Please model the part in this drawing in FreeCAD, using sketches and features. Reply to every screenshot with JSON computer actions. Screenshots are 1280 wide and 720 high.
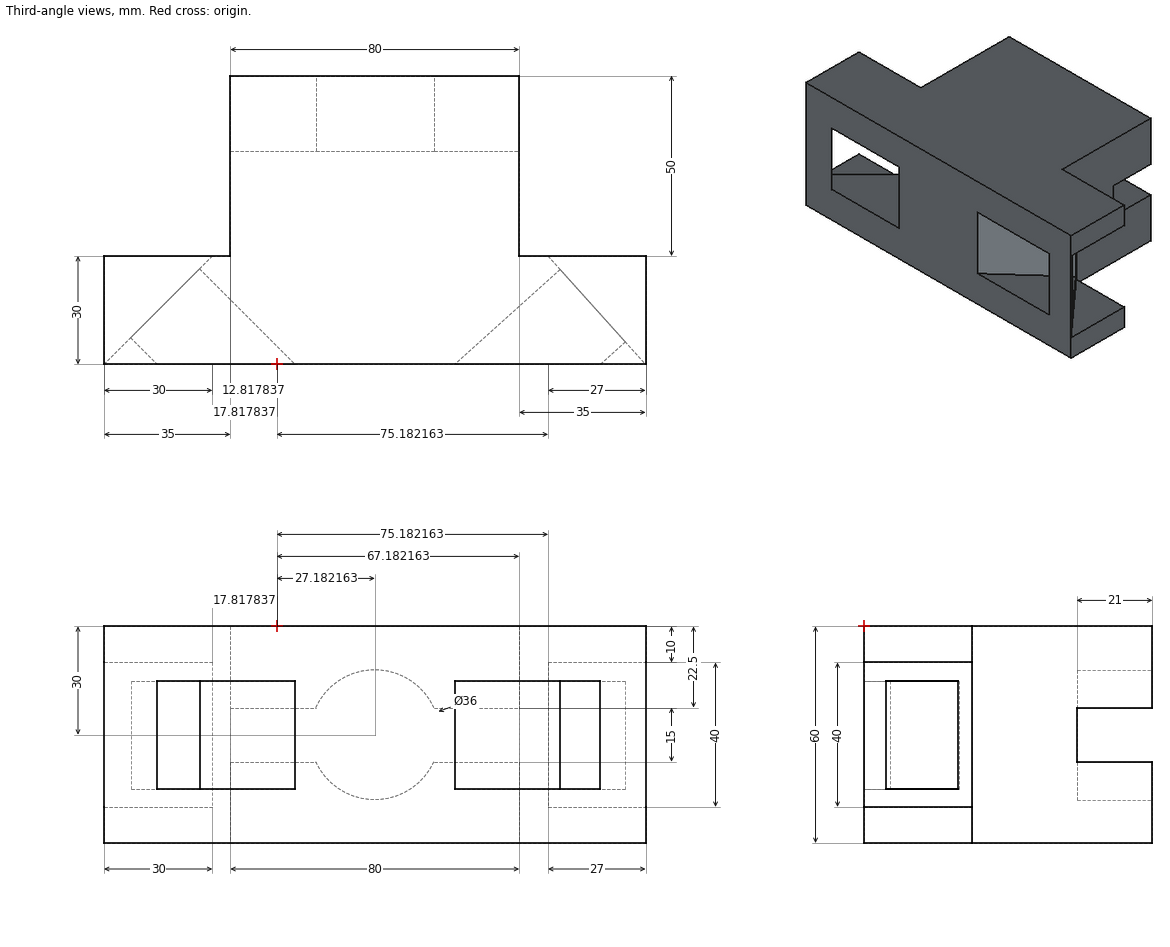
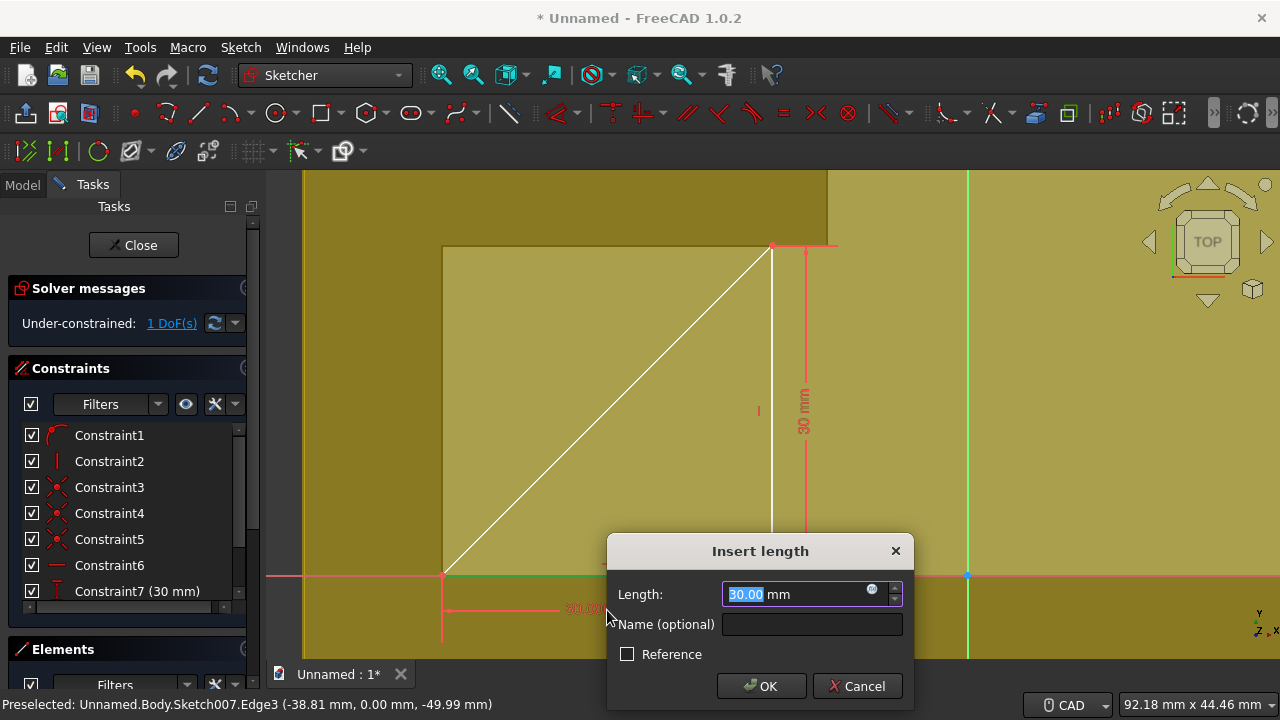
{"action": "type", "text": "30"}
{"action": "key", "text": "Return"}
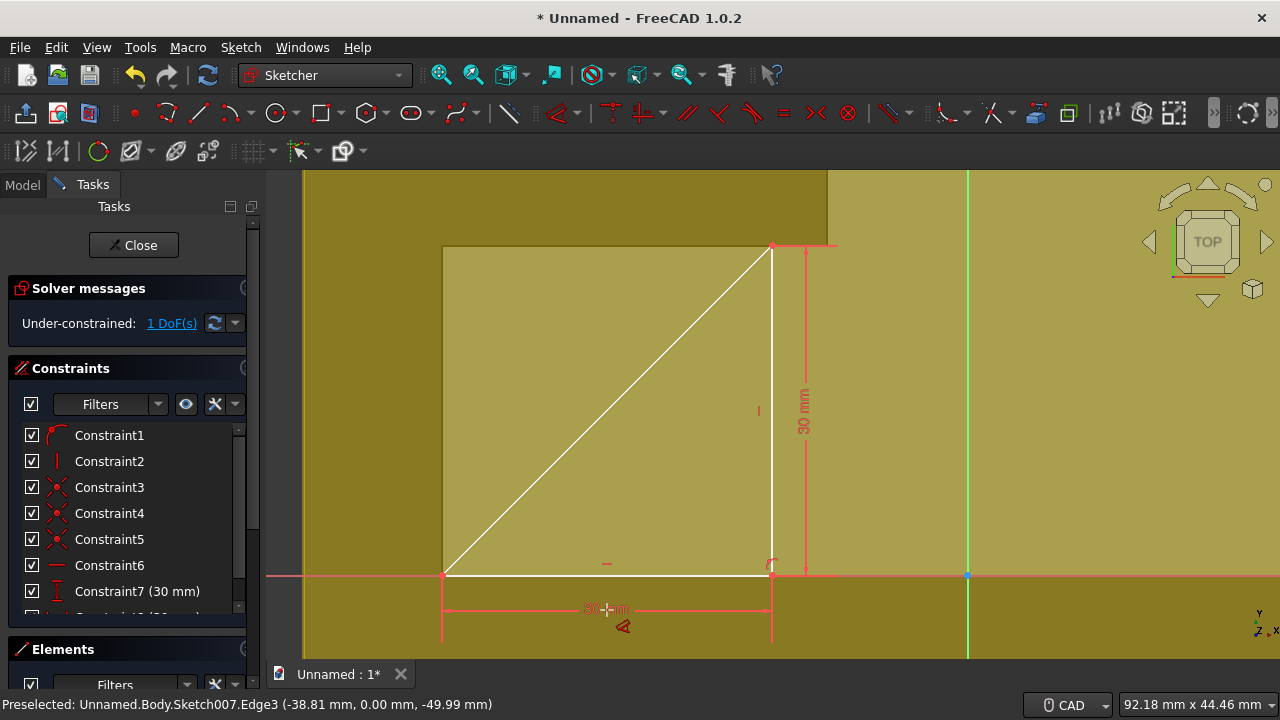
{"action": "left_click", "coordinate": [772, 576]}
{"action": "left_click", "coordinate": [870, 610]}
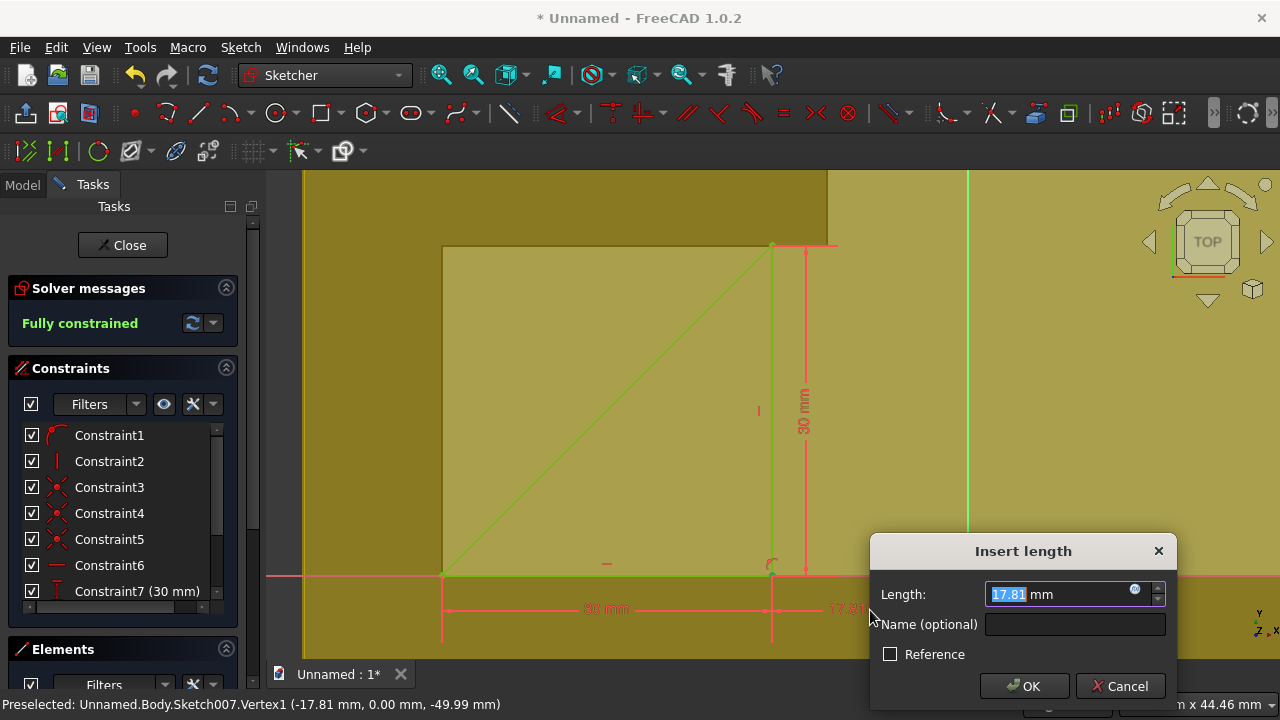
{"action": "type", "text": "17.817837"}
{"action": "key", "text": "Return"}
{"action": "key", "text": "Escape"}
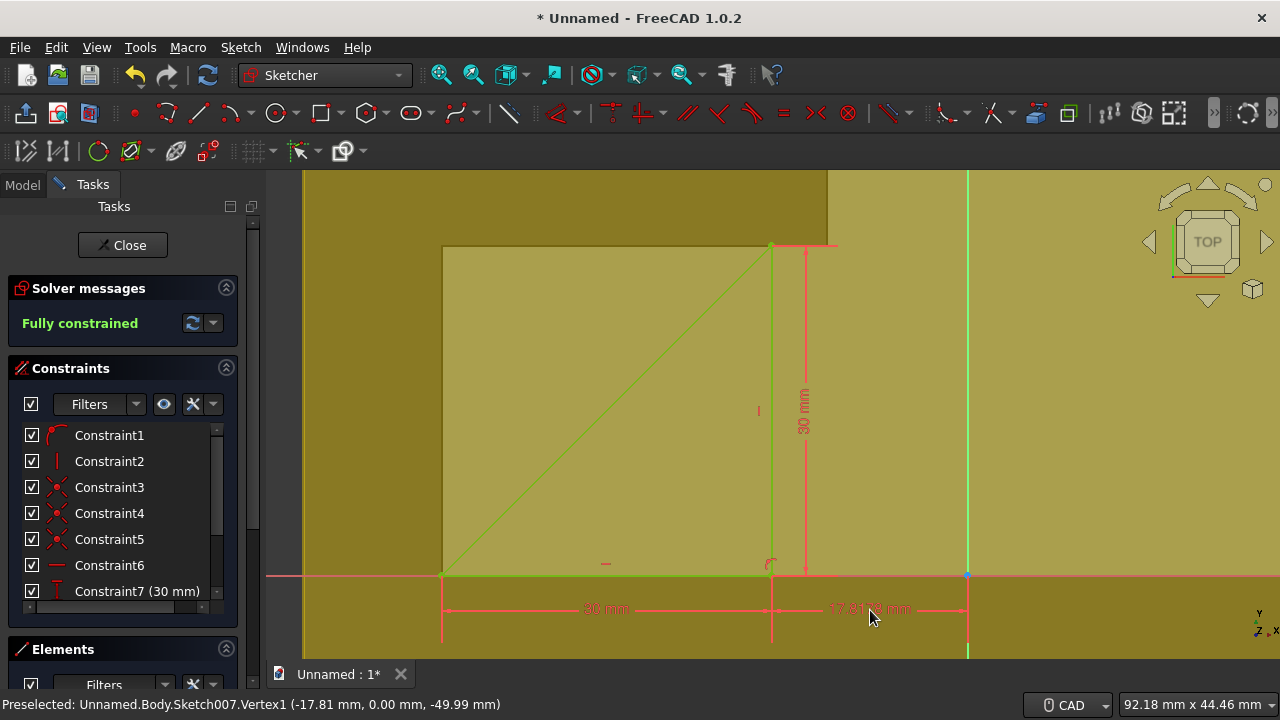
{"action": "left_click", "coordinate": [123, 245]}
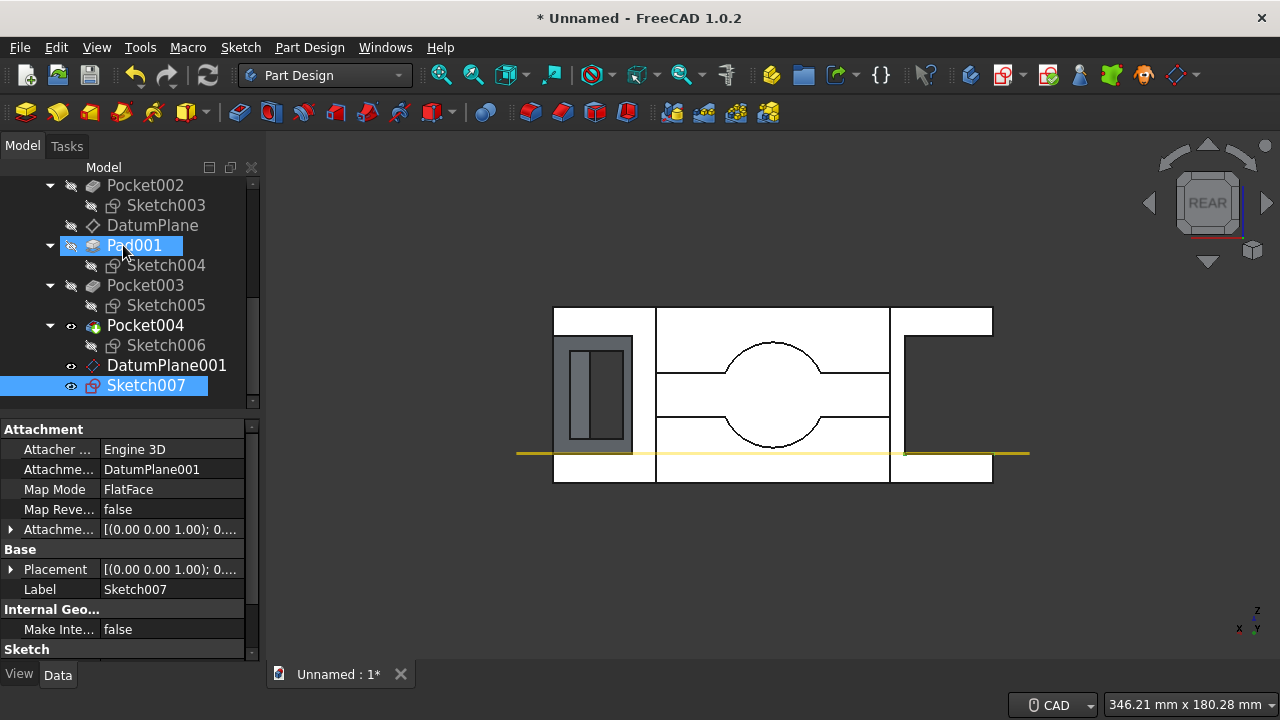
{"action": "left_click", "coordinate": [26, 112]}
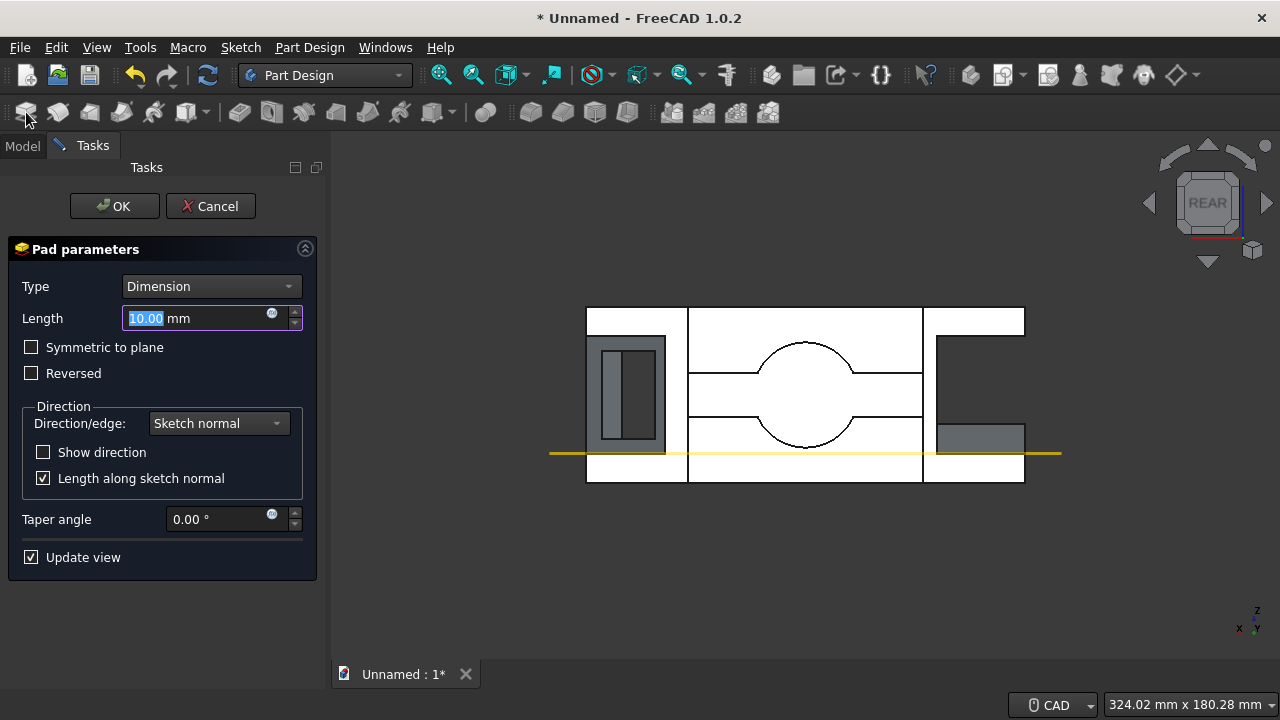
{"action": "type", "text": "40"}
{"action": "key", "text": "Tab"}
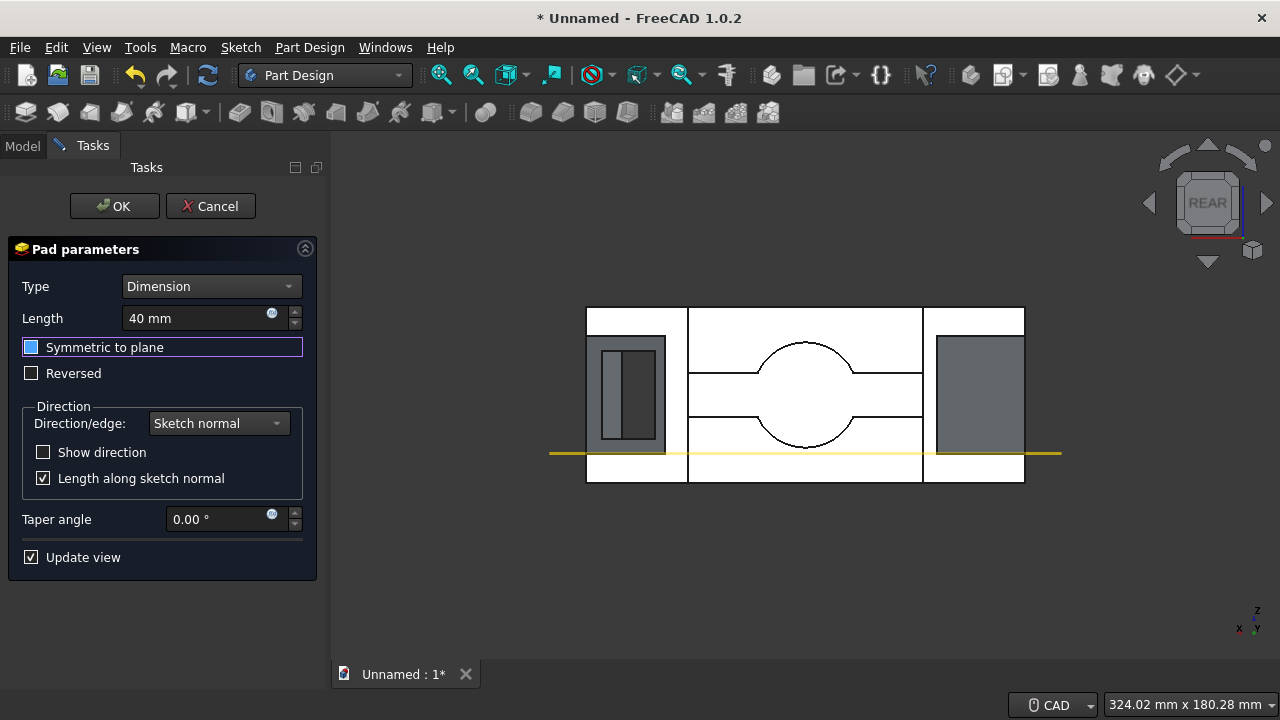
{"action": "left_click", "coordinate": [115, 206]}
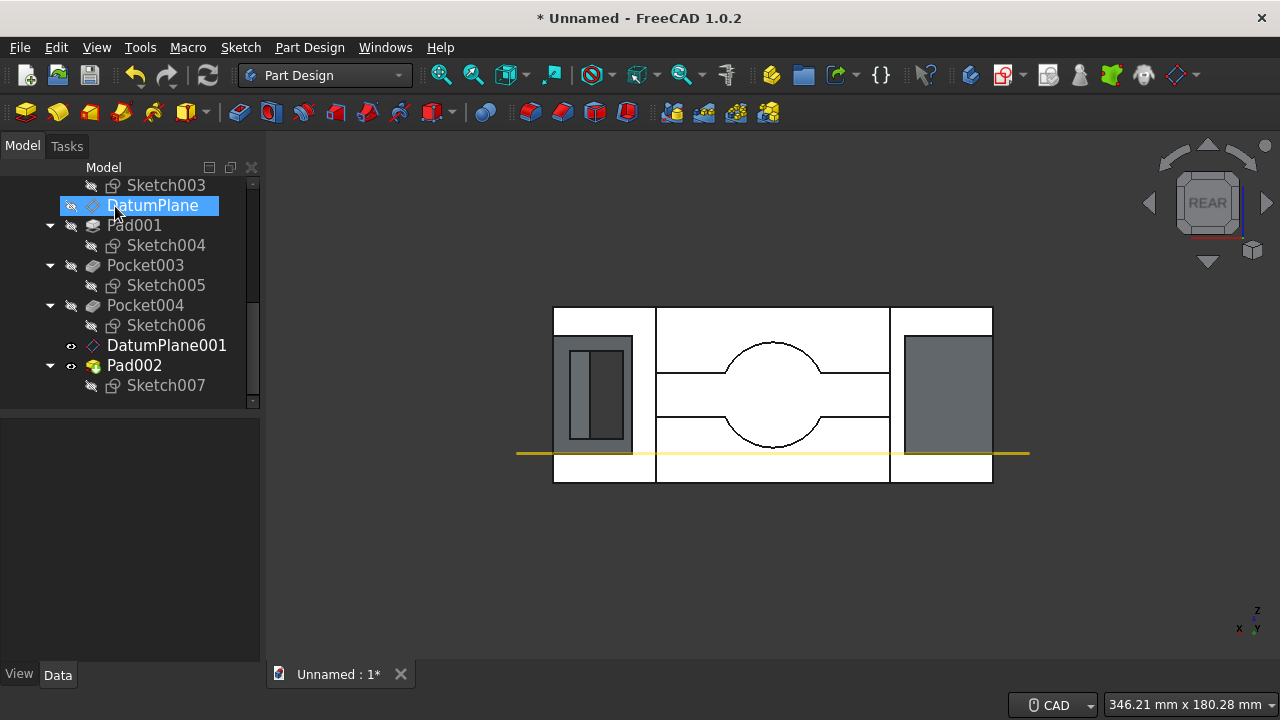
{"action": "left_click", "coordinate": [116, 346]}
{"action": "key", "text": "space"}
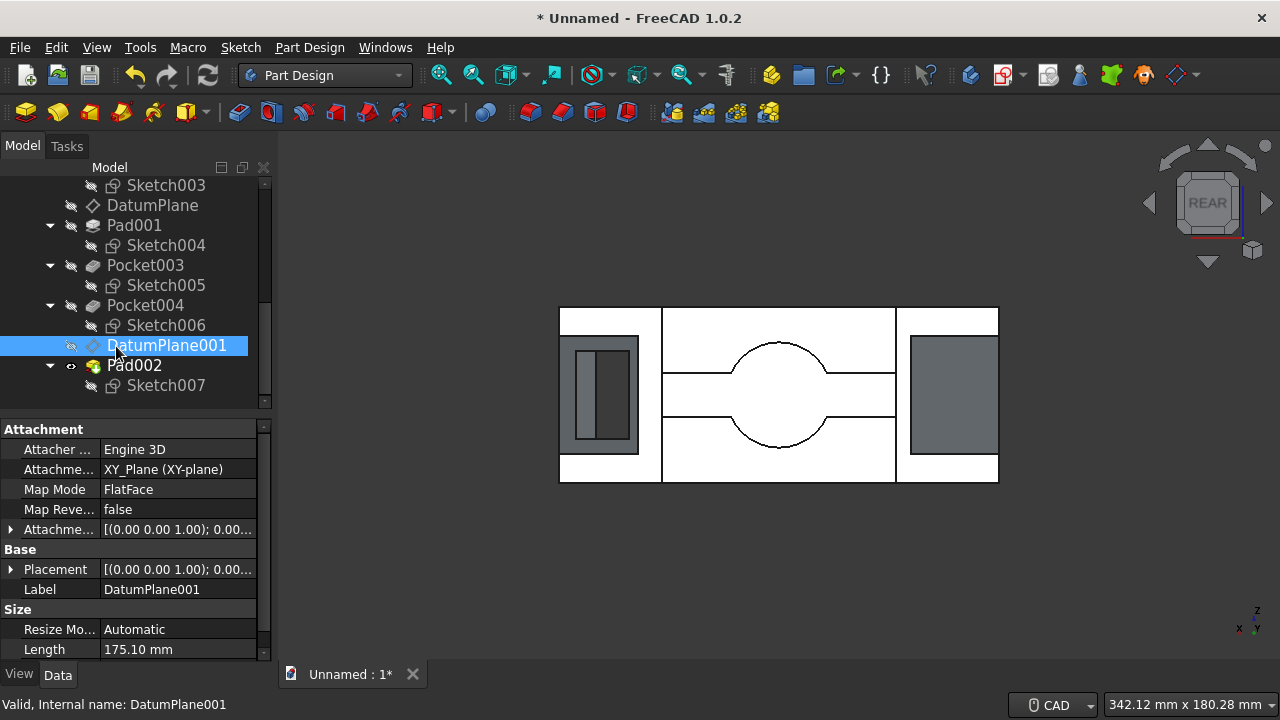
{"action": "left_click", "coordinate": [442, 76]}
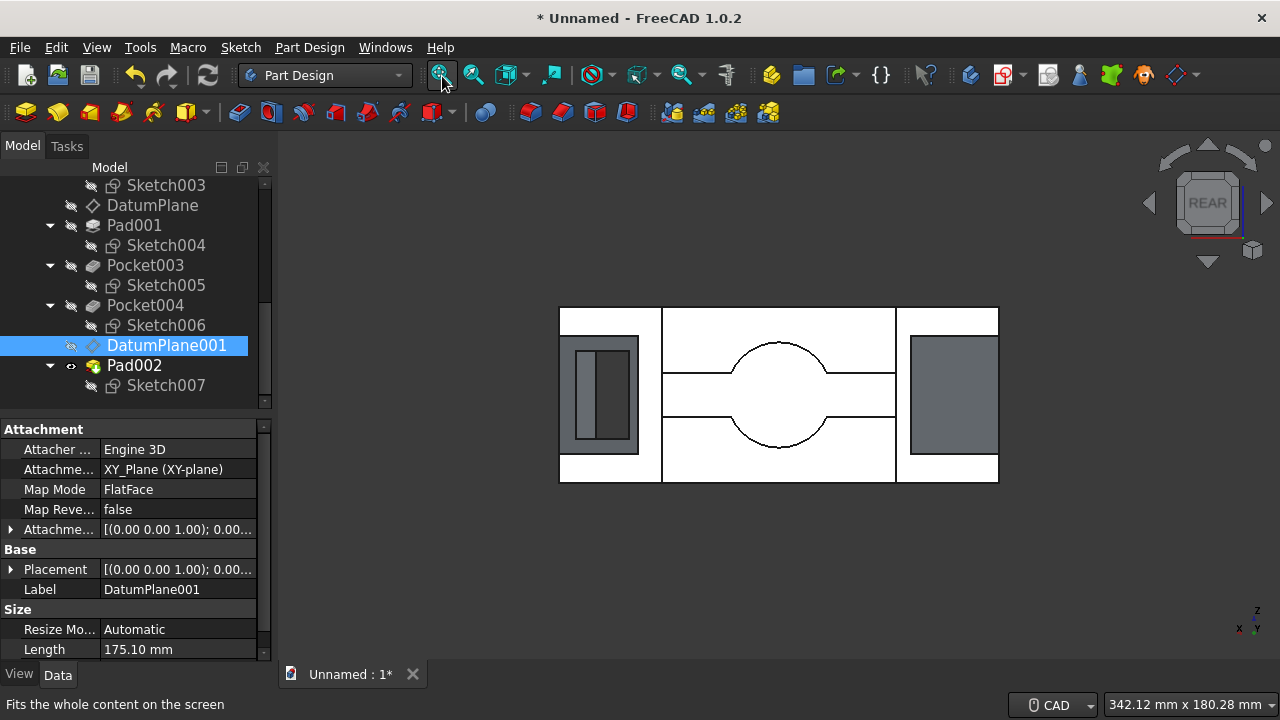
{"action": "left_click", "coordinate": [955, 394]}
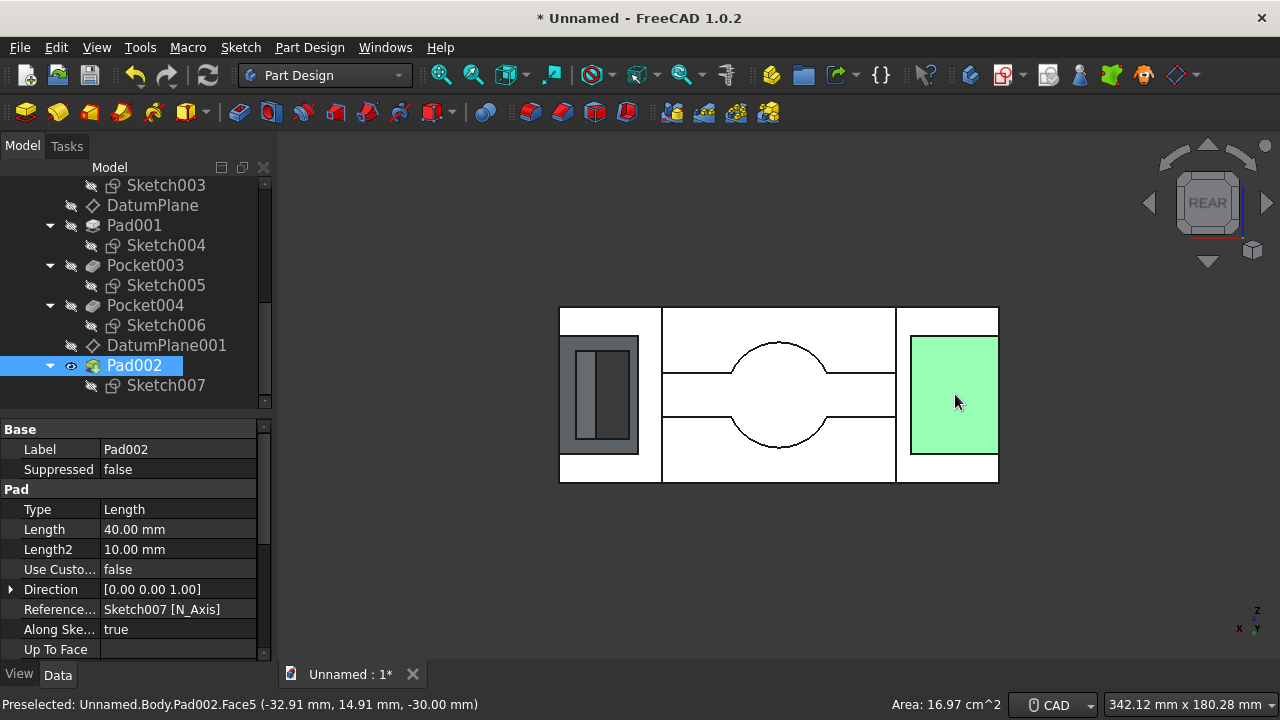
{"action": "left_click", "coordinate": [1004, 76]}